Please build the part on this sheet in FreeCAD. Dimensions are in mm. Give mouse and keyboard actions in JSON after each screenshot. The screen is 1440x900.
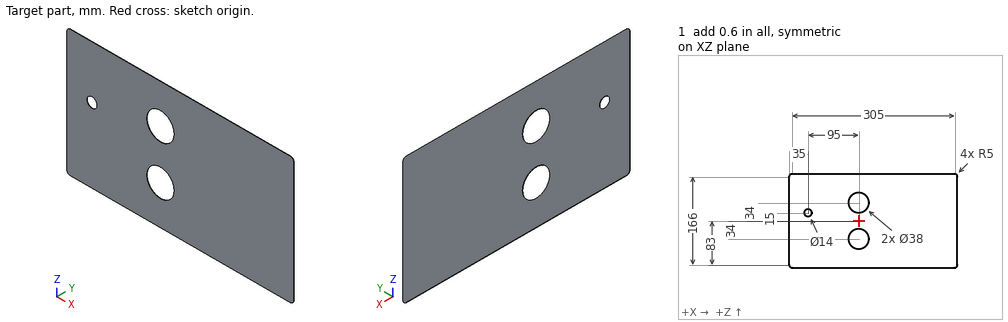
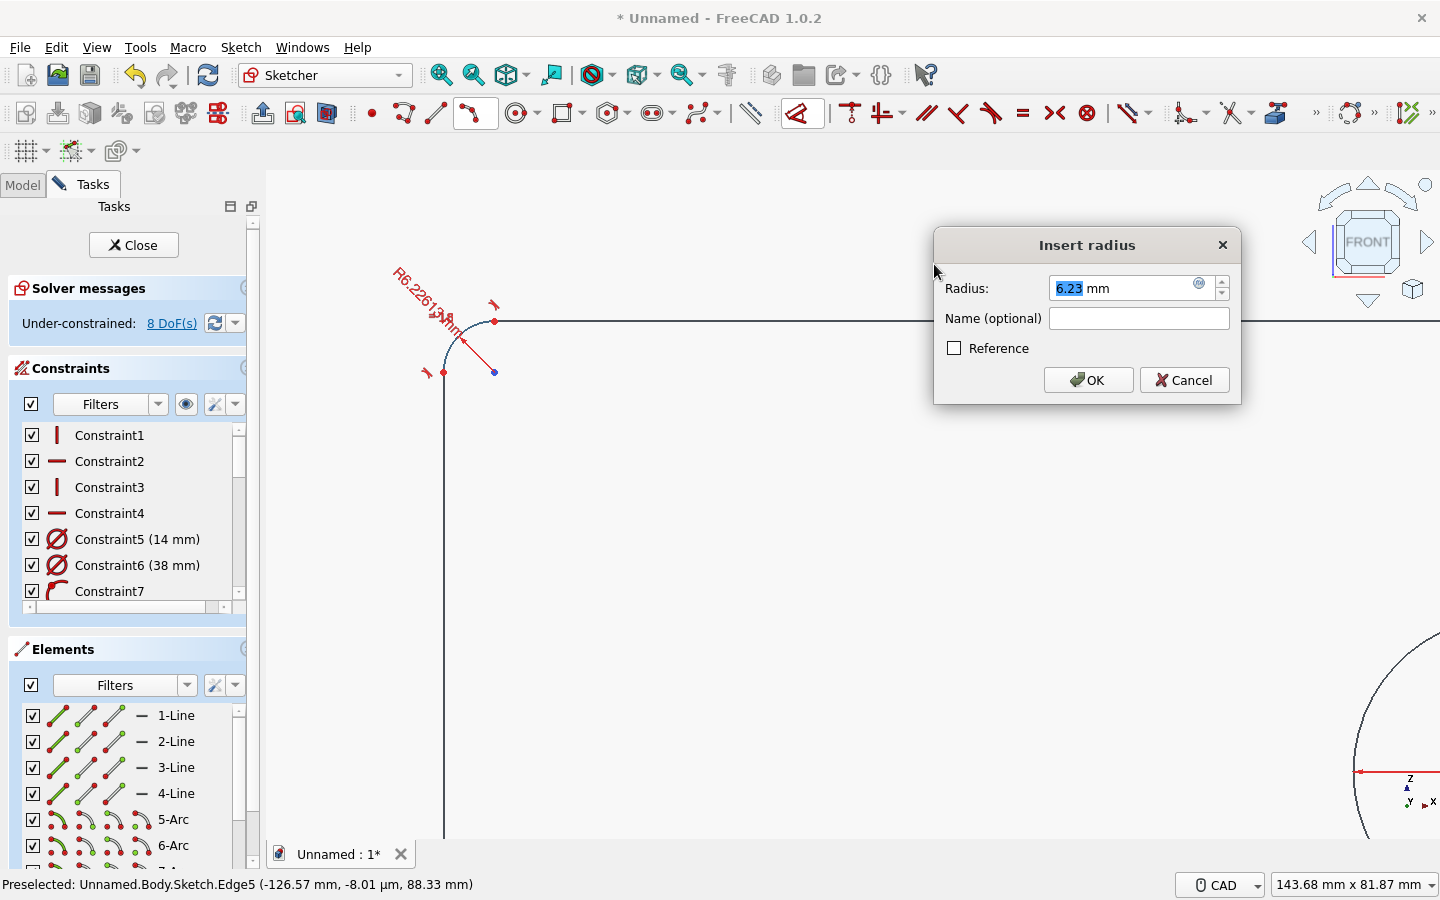
{"action": "type", "text": "5"}
{"action": "key", "text": "Return"}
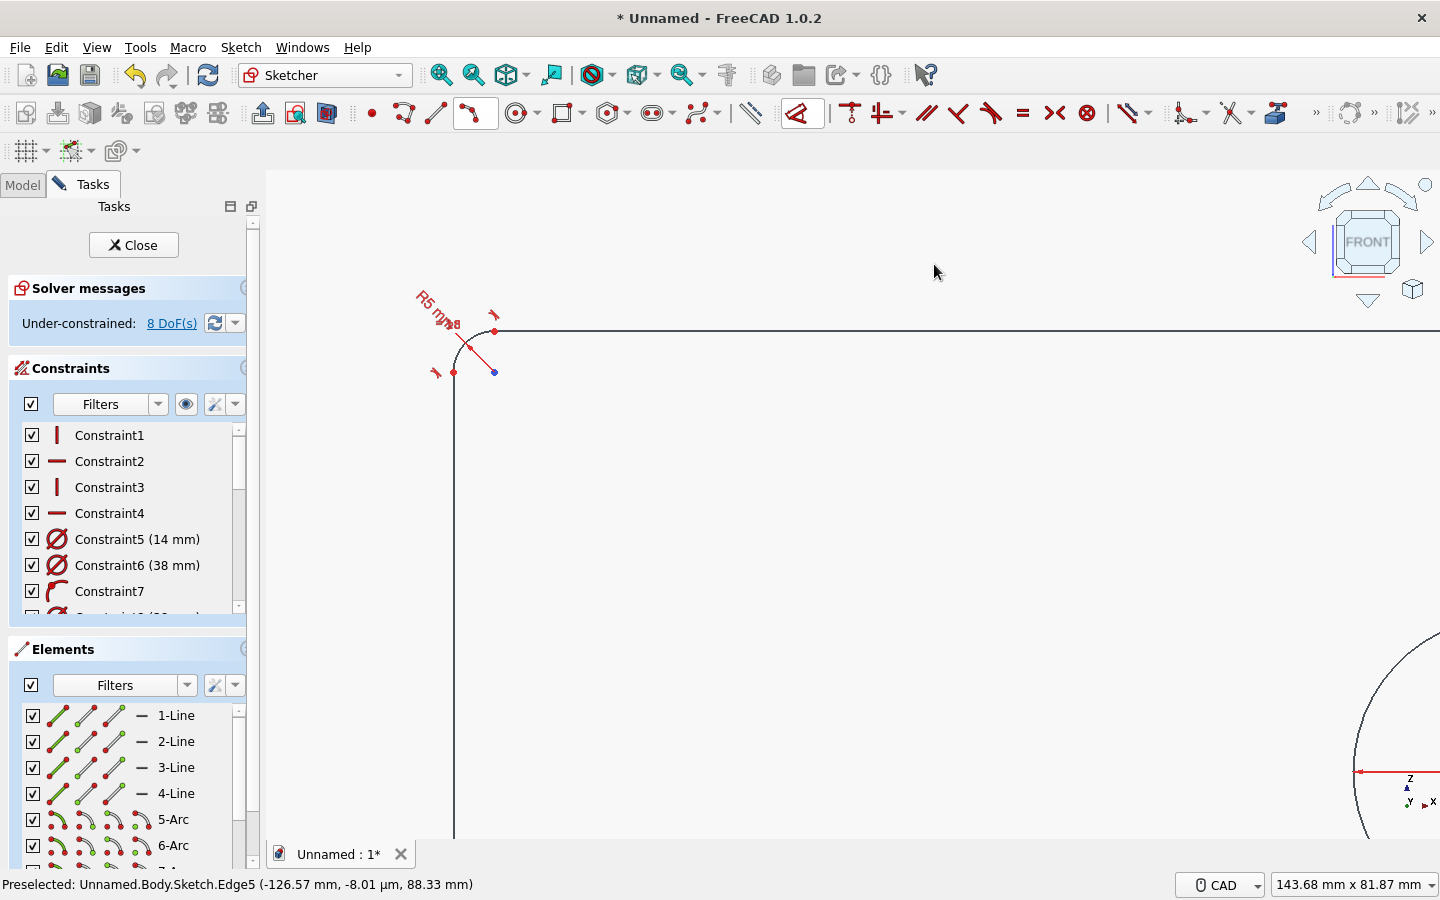
{"action": "scroll", "coordinate": [474, 327], "scroll_direction": "down", "scroll_amount": 7}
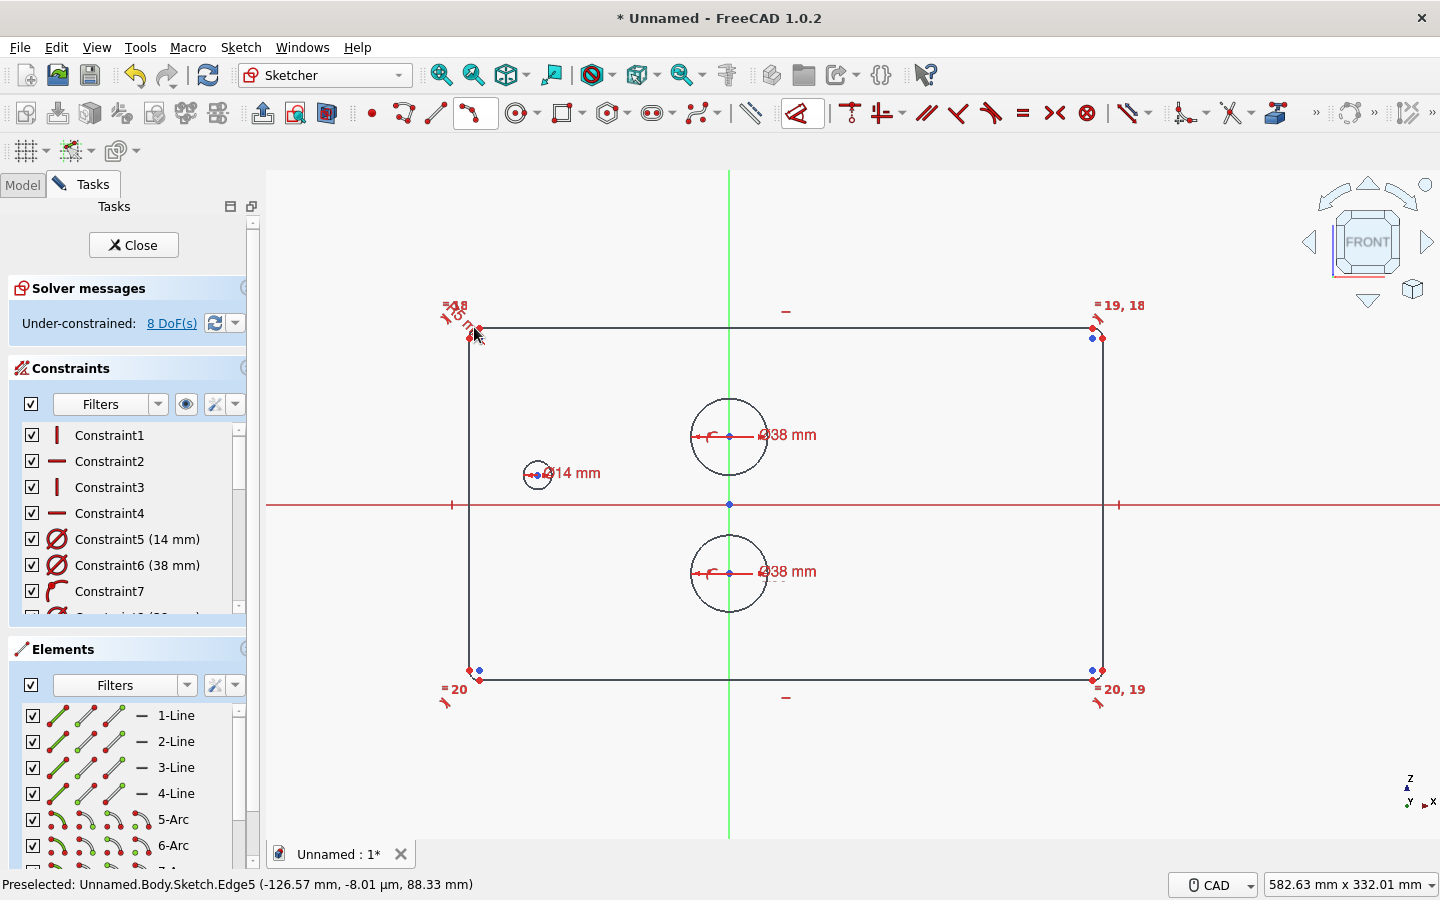
{"action": "left_click", "coordinate": [538, 475]}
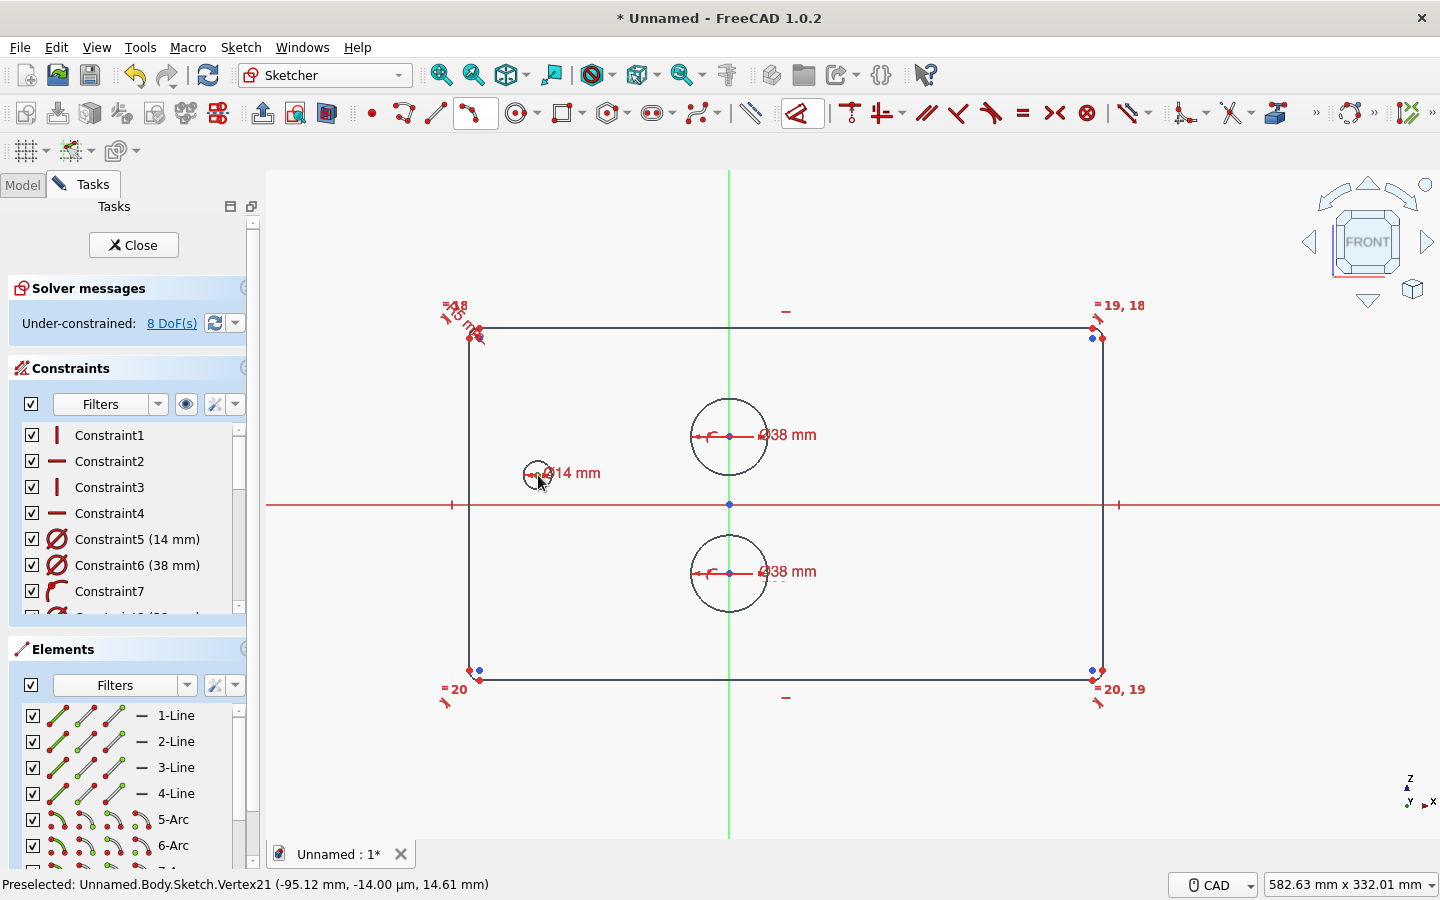
{"action": "key", "text": "l"}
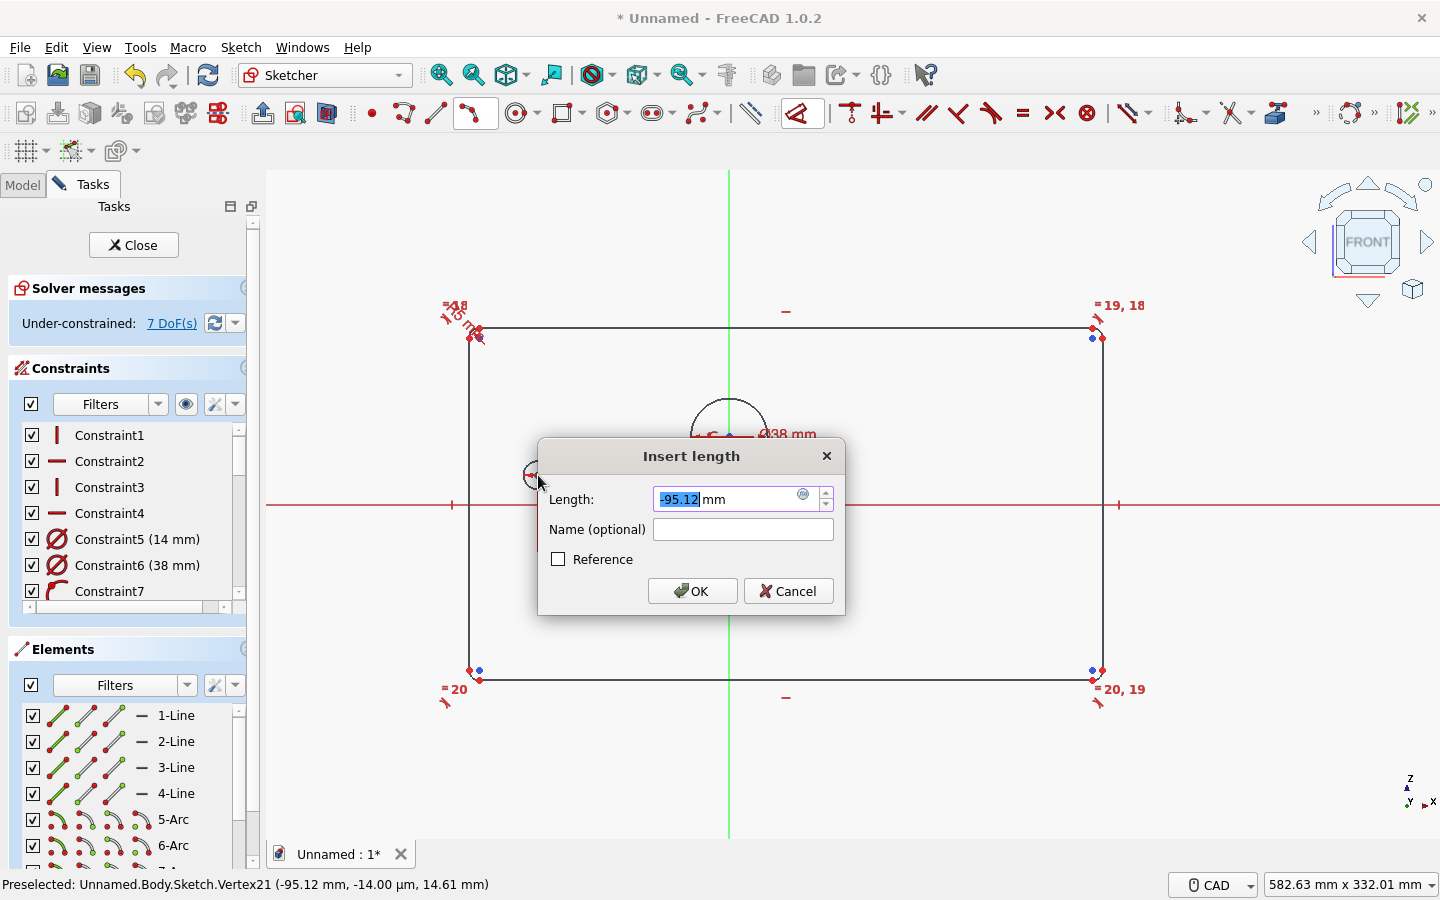
{"action": "type", "text": "-95"}
{"action": "key", "text": "Return"}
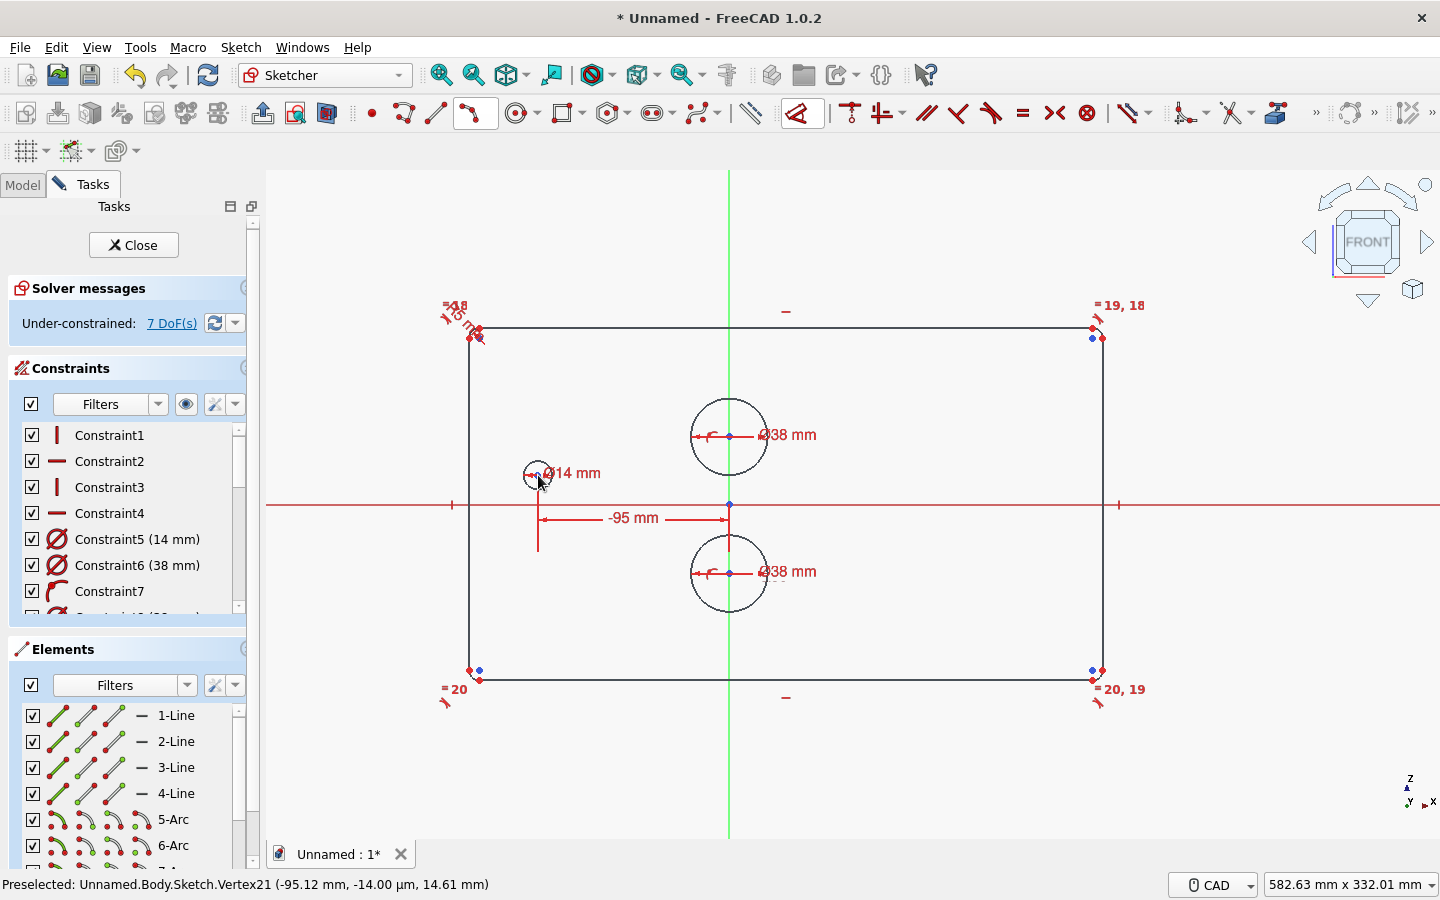
{"action": "scroll", "coordinate": [538, 475], "scroll_direction": "up", "scroll_amount": 2}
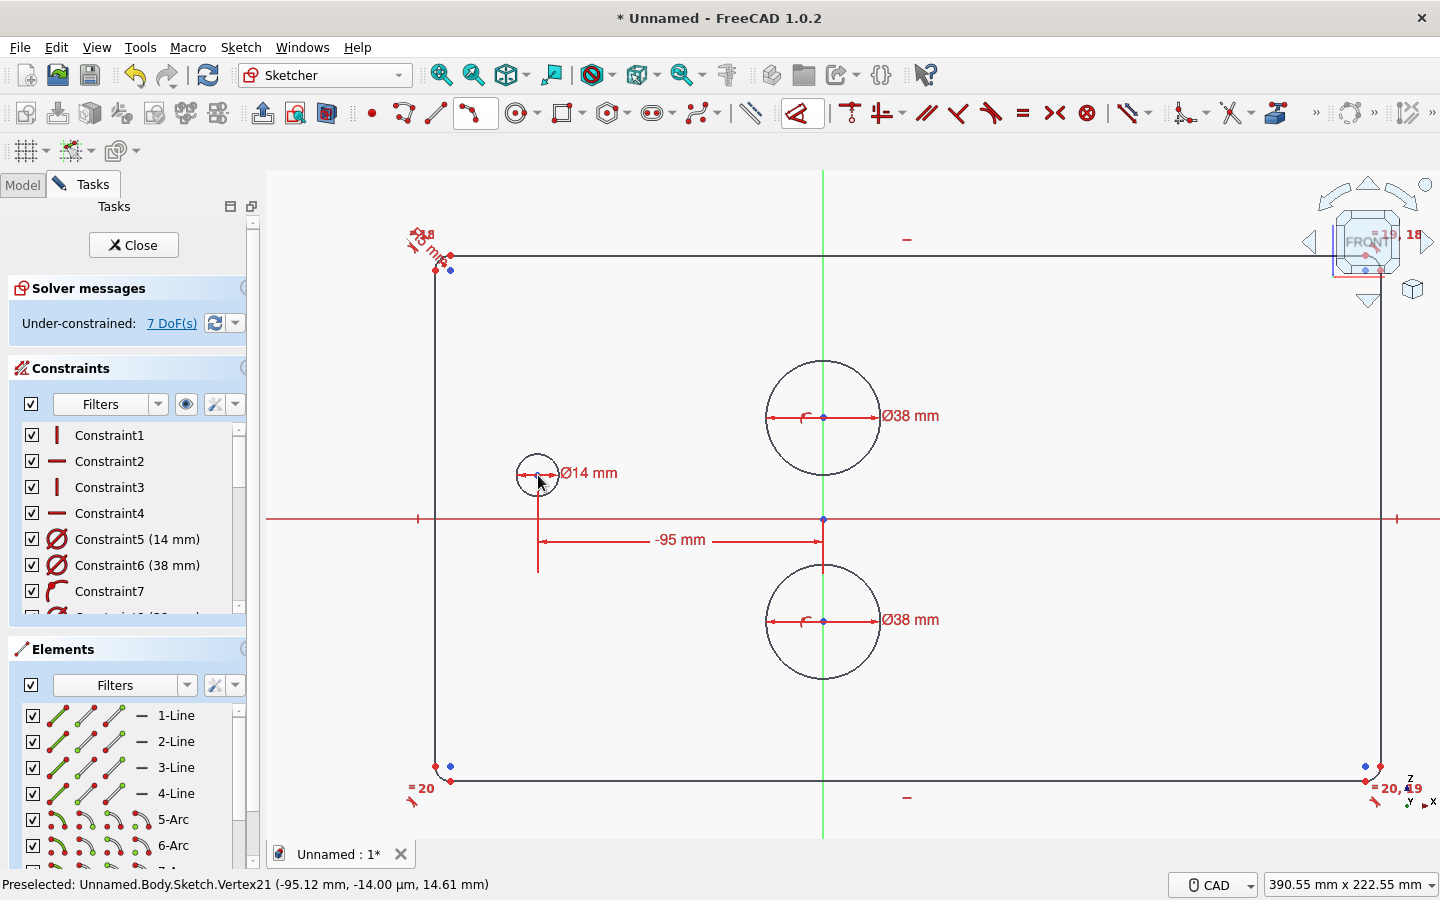
{"action": "left_click", "coordinate": [538, 475]}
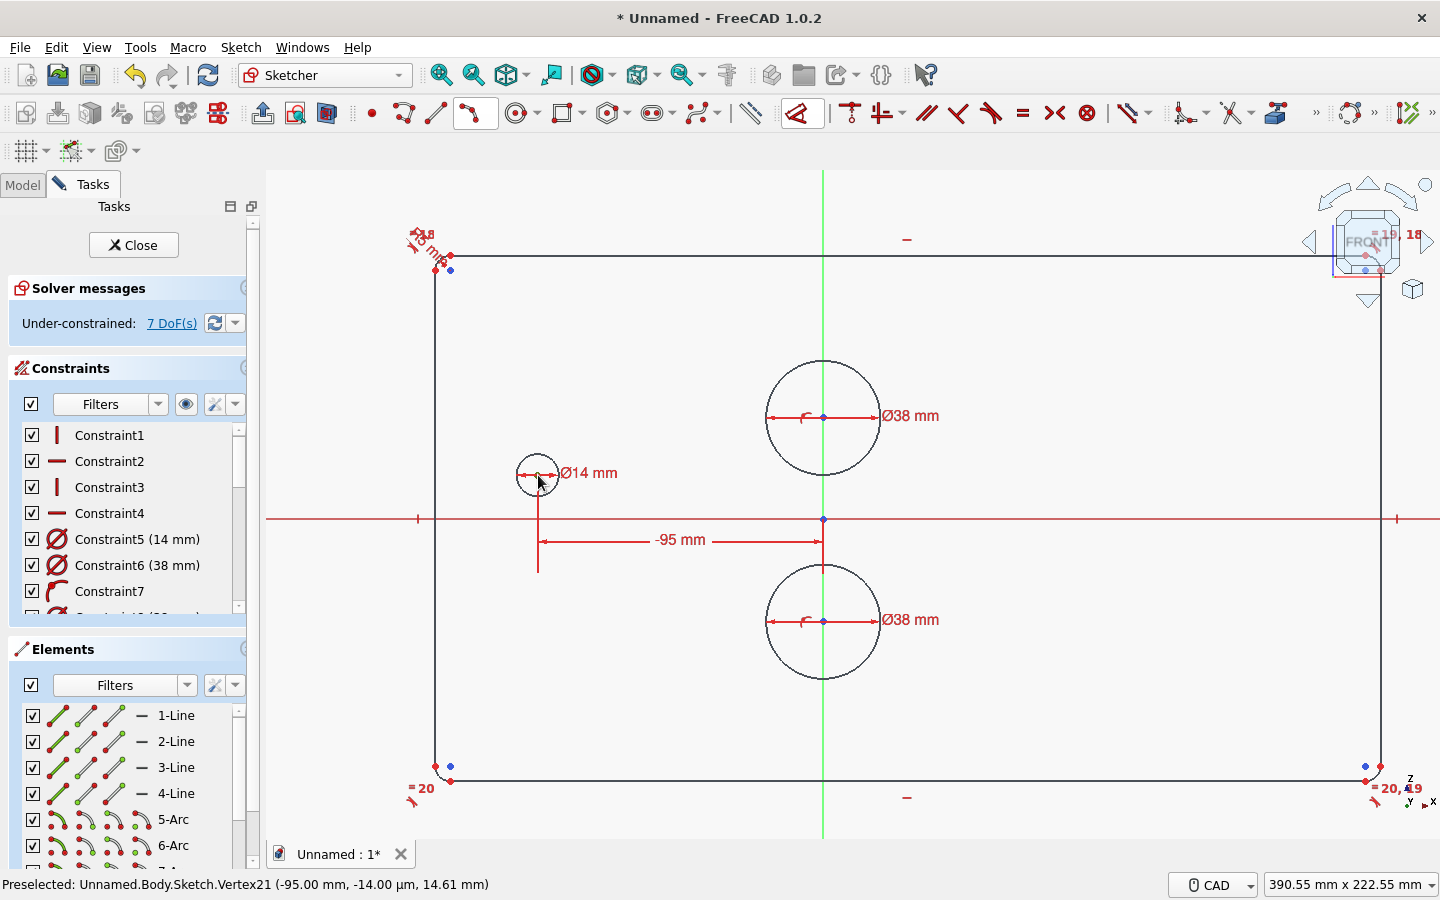
{"action": "left_click", "coordinate": [818, 114]}